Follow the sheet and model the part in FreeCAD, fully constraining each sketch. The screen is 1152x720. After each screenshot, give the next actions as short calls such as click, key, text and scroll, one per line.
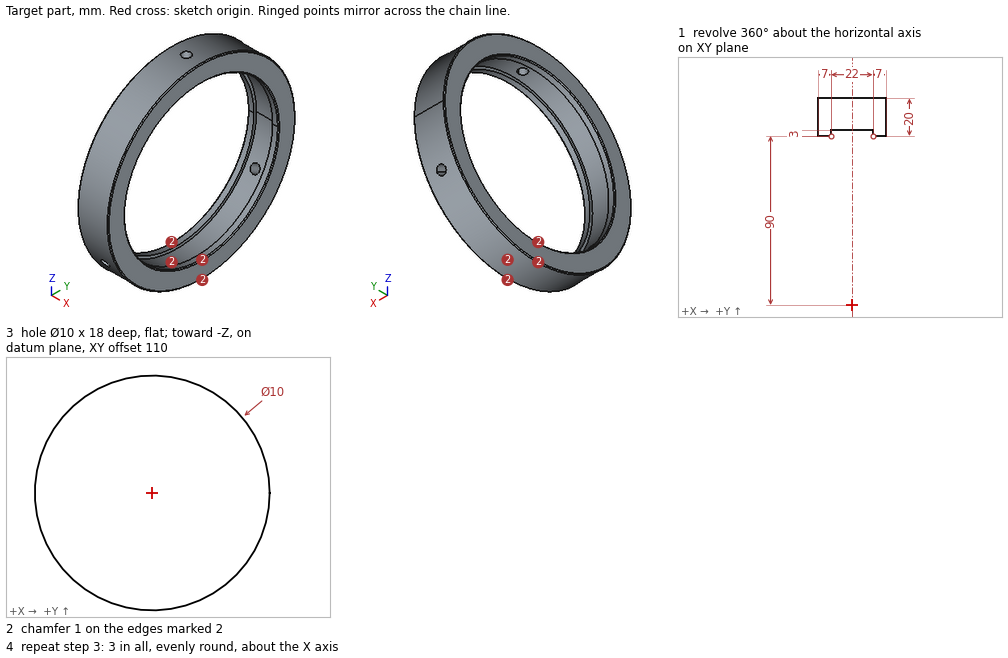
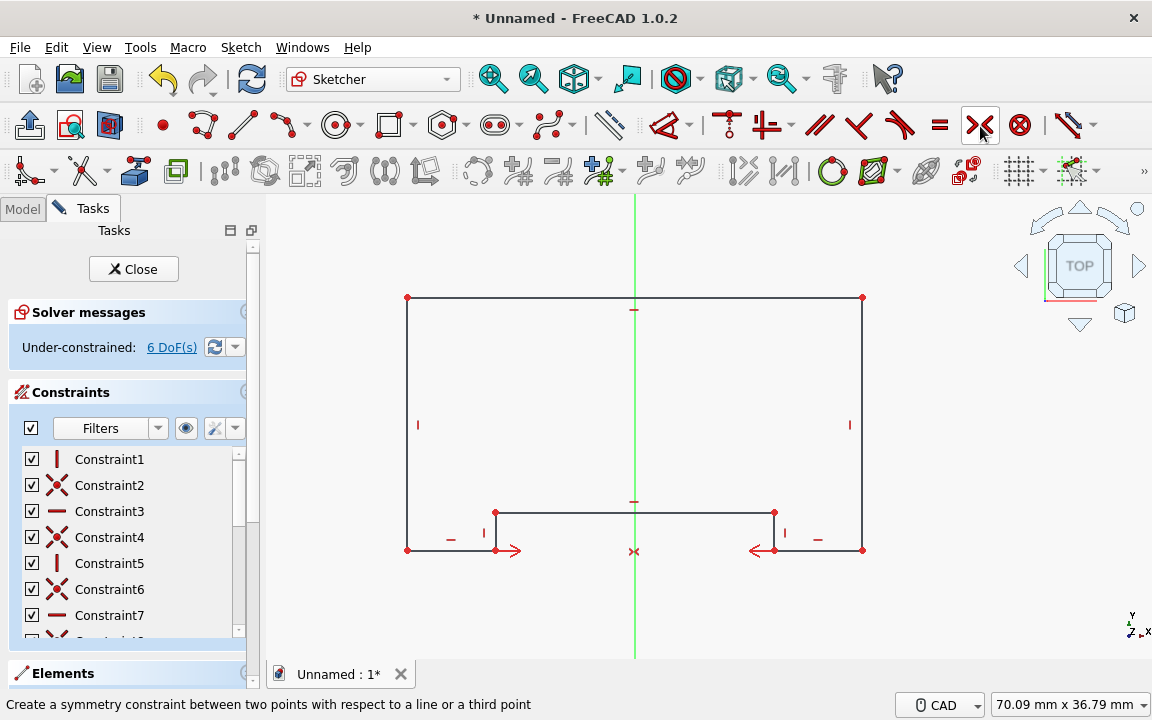
click(496, 540)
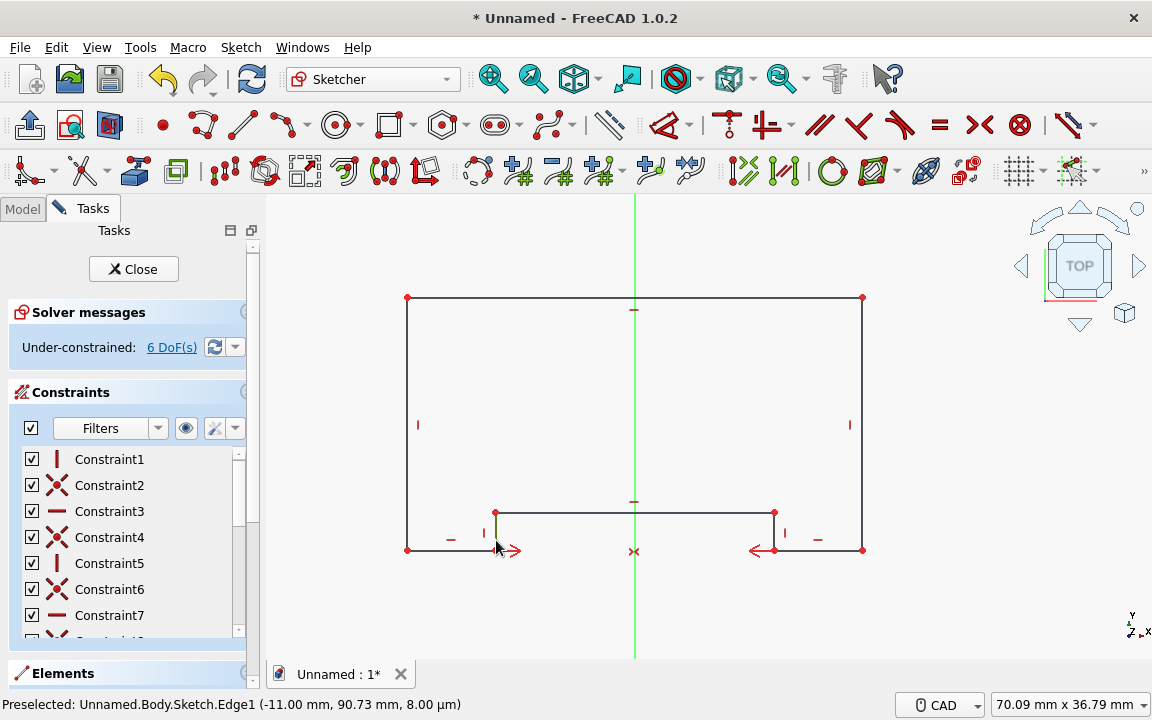
key(i)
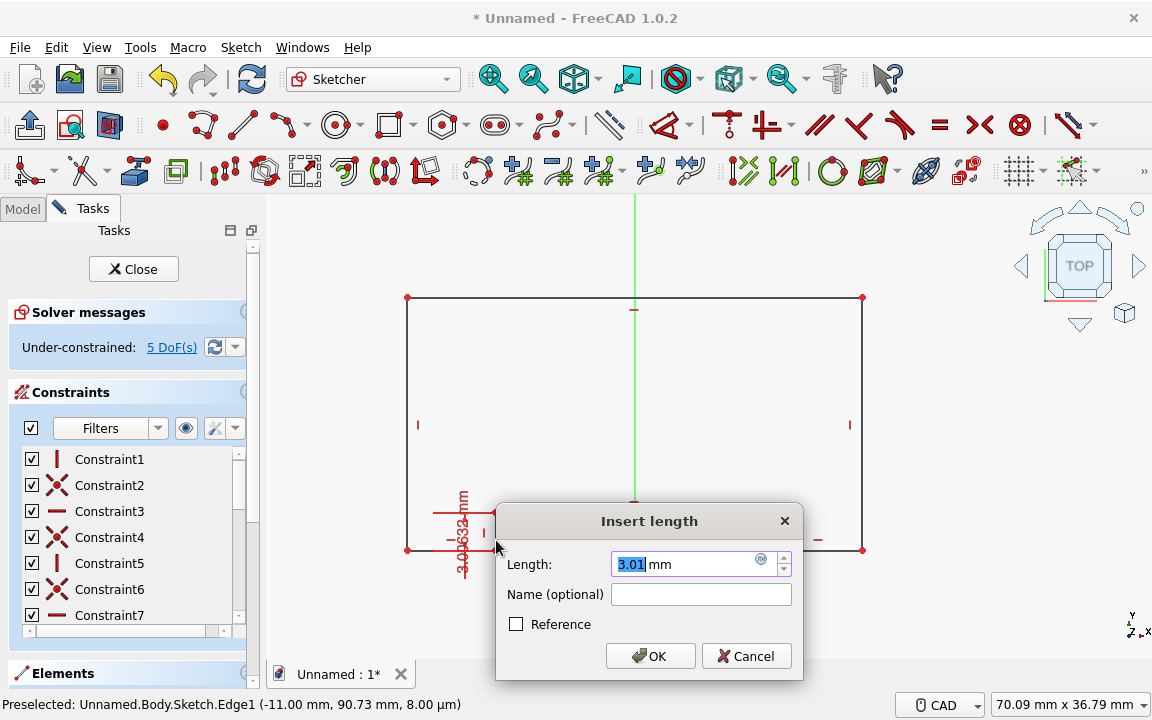
text(3)
key(Return)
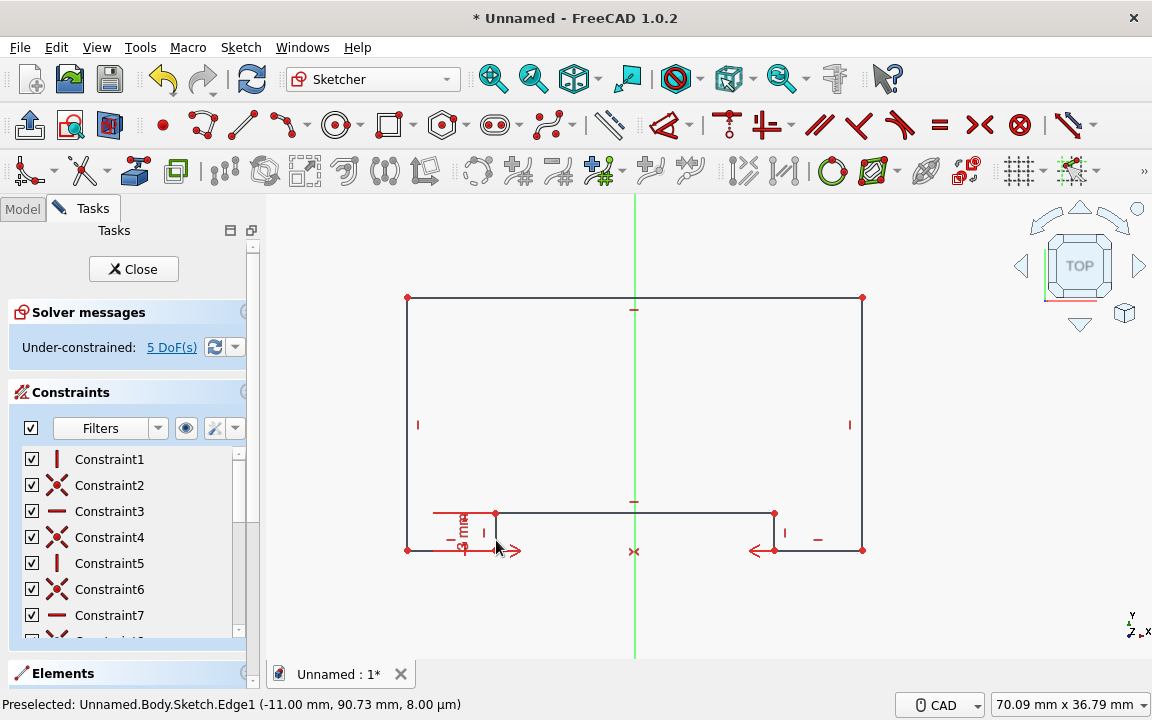
click(800, 551)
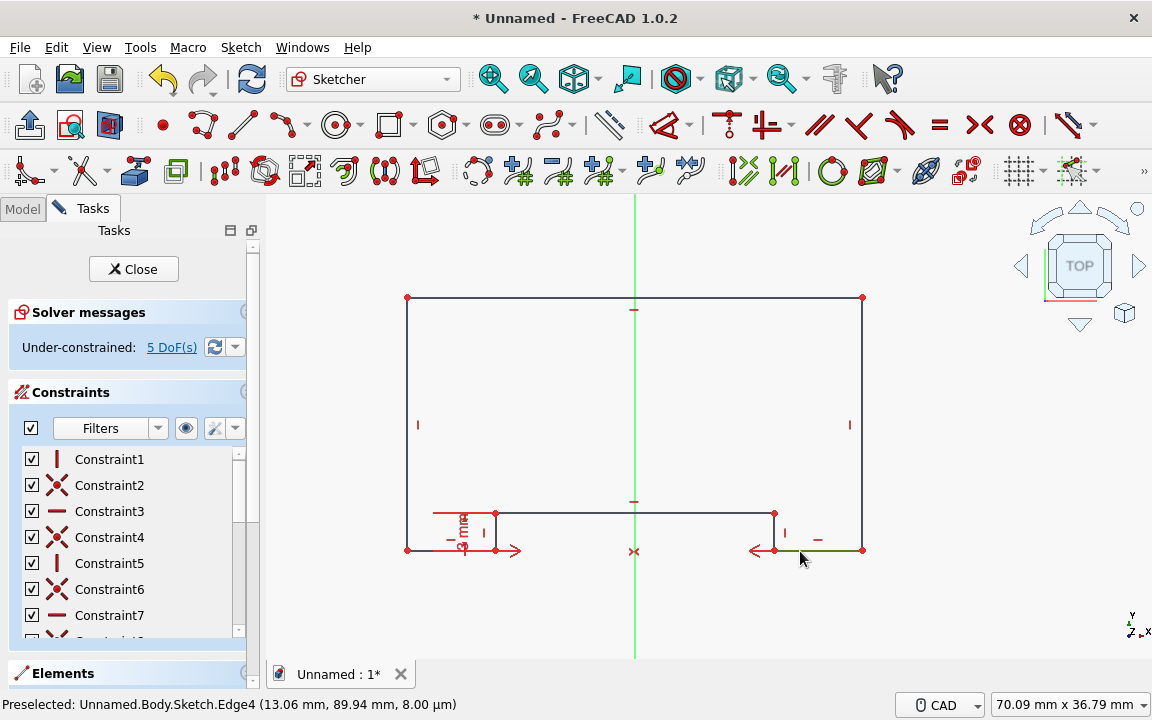
key(l)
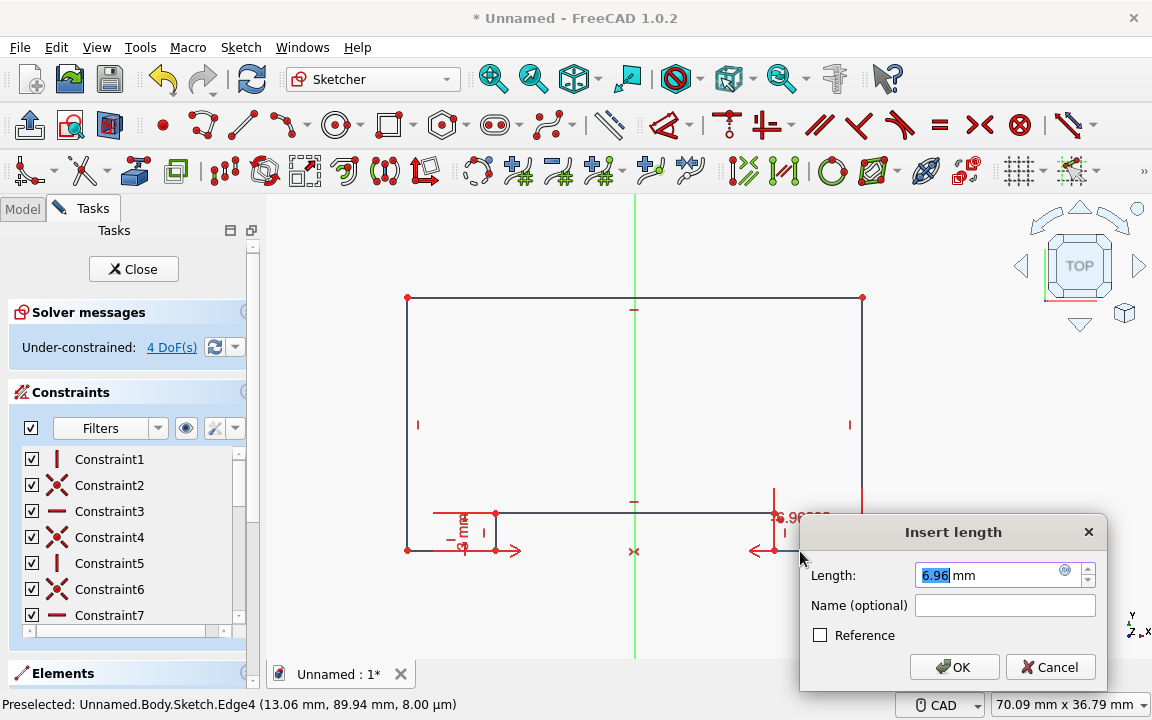
text(7)
key(Return)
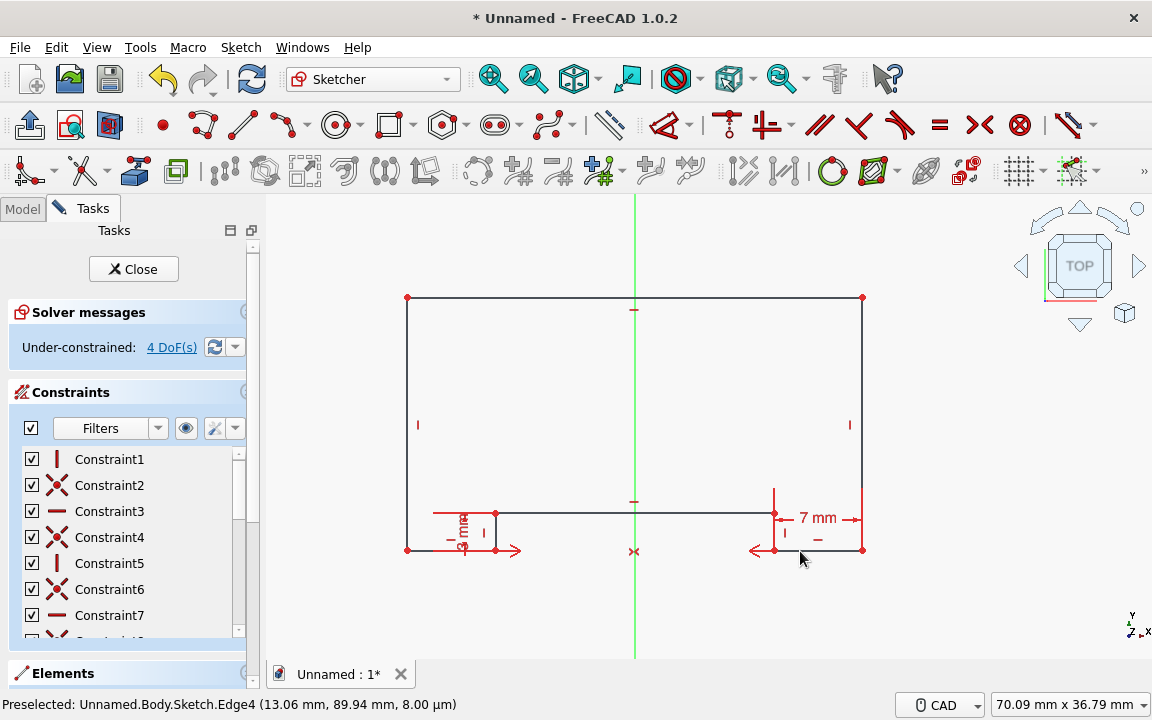
click(434, 551)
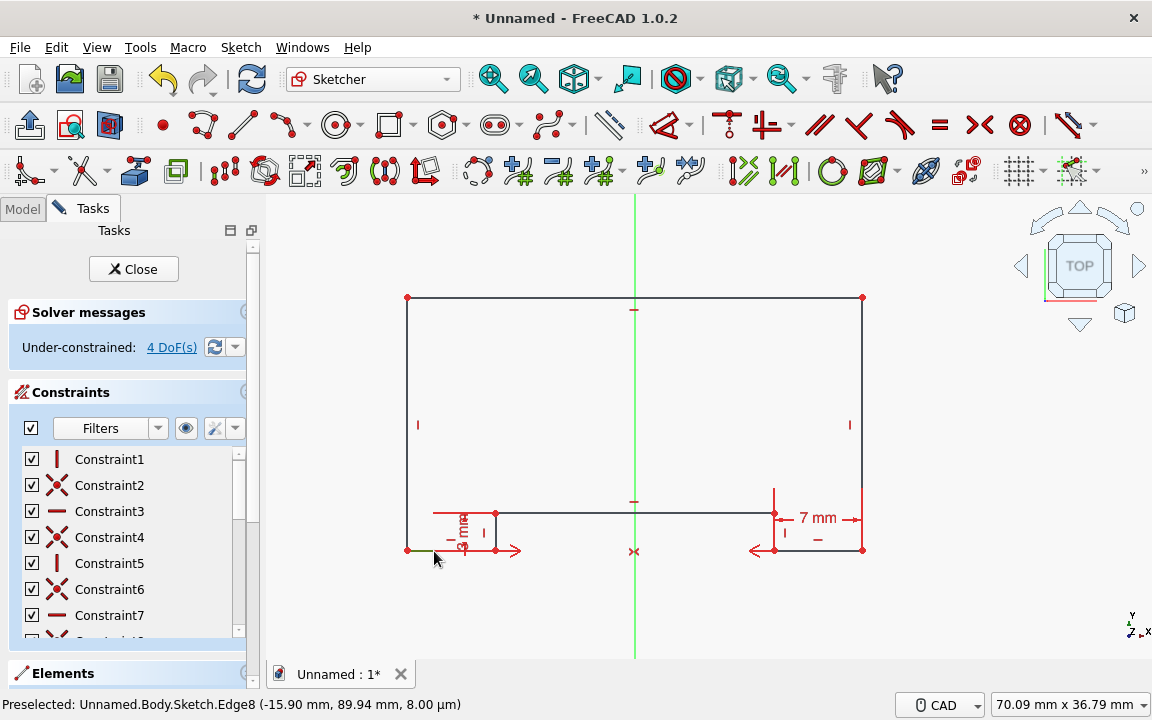
key(l)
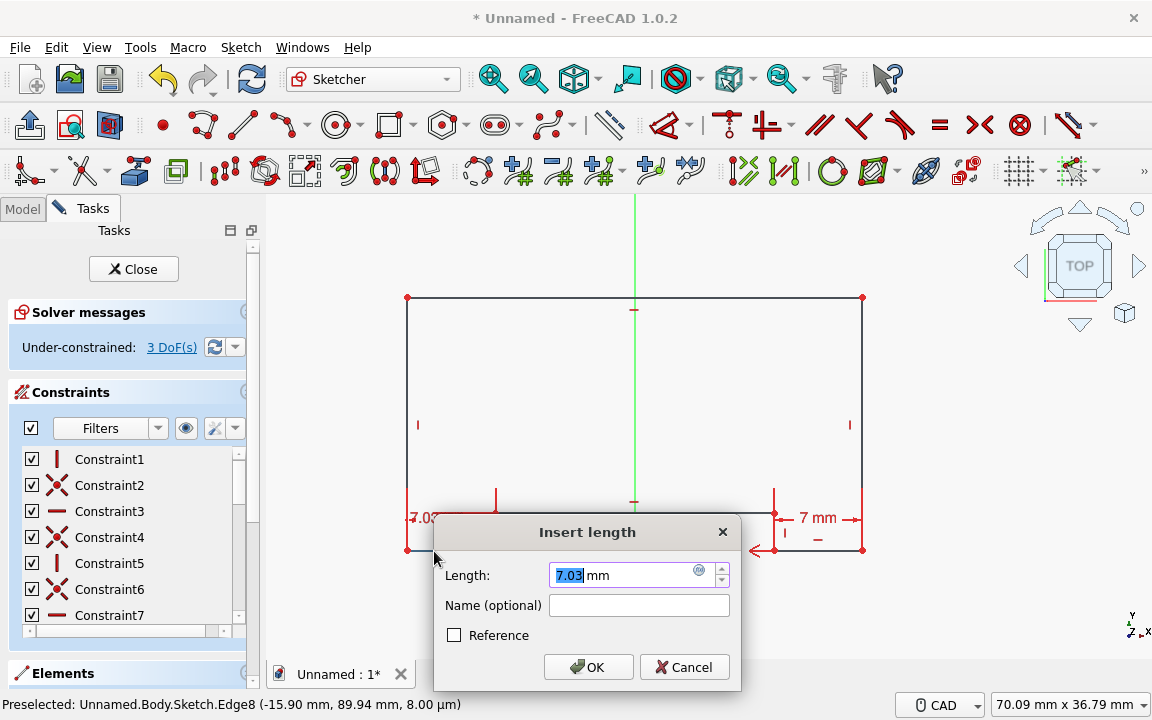
text(7)
key(Return)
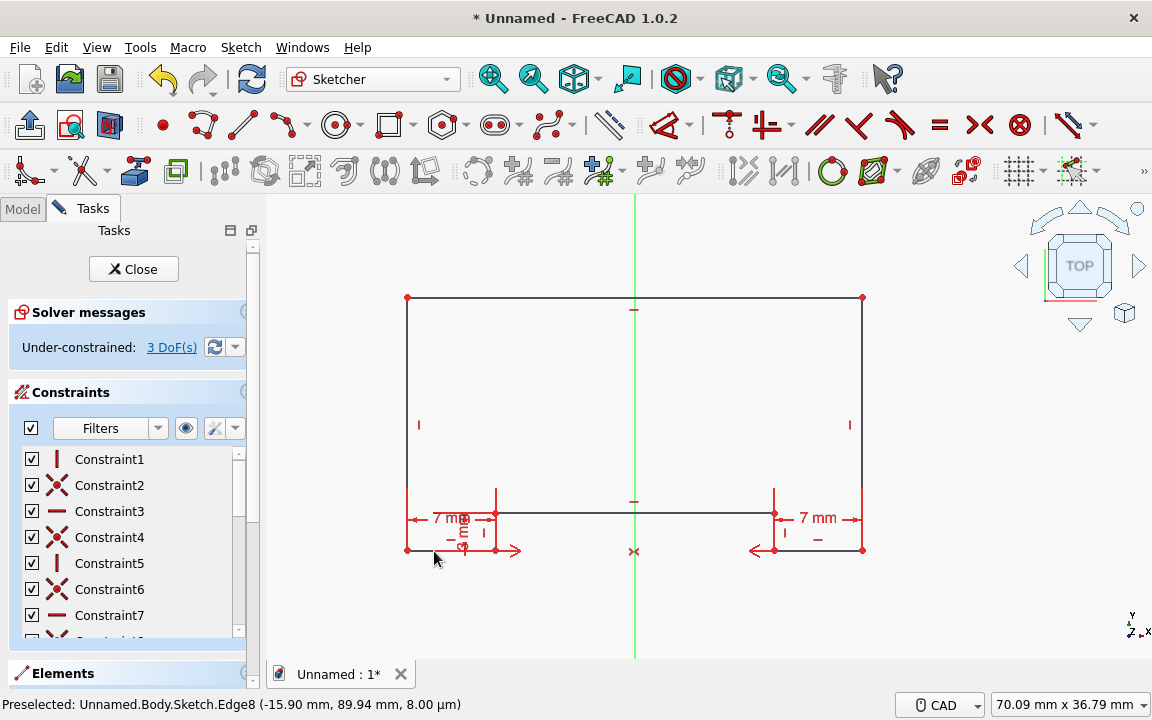
click(579, 513)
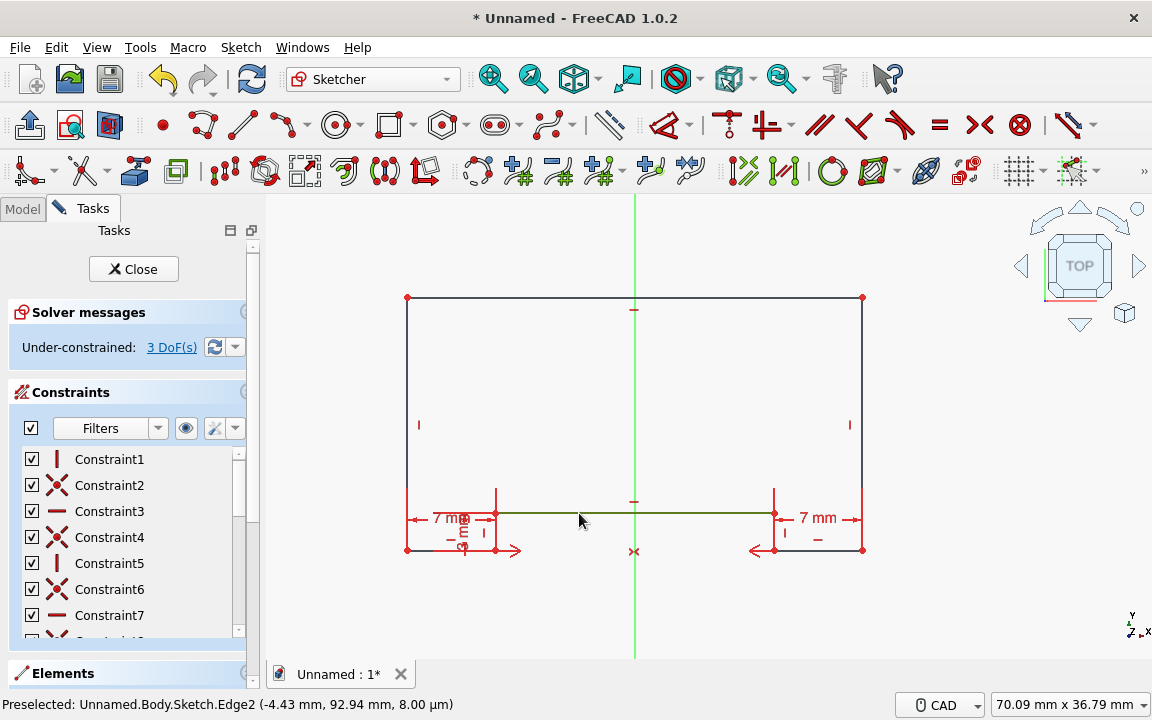
key(l)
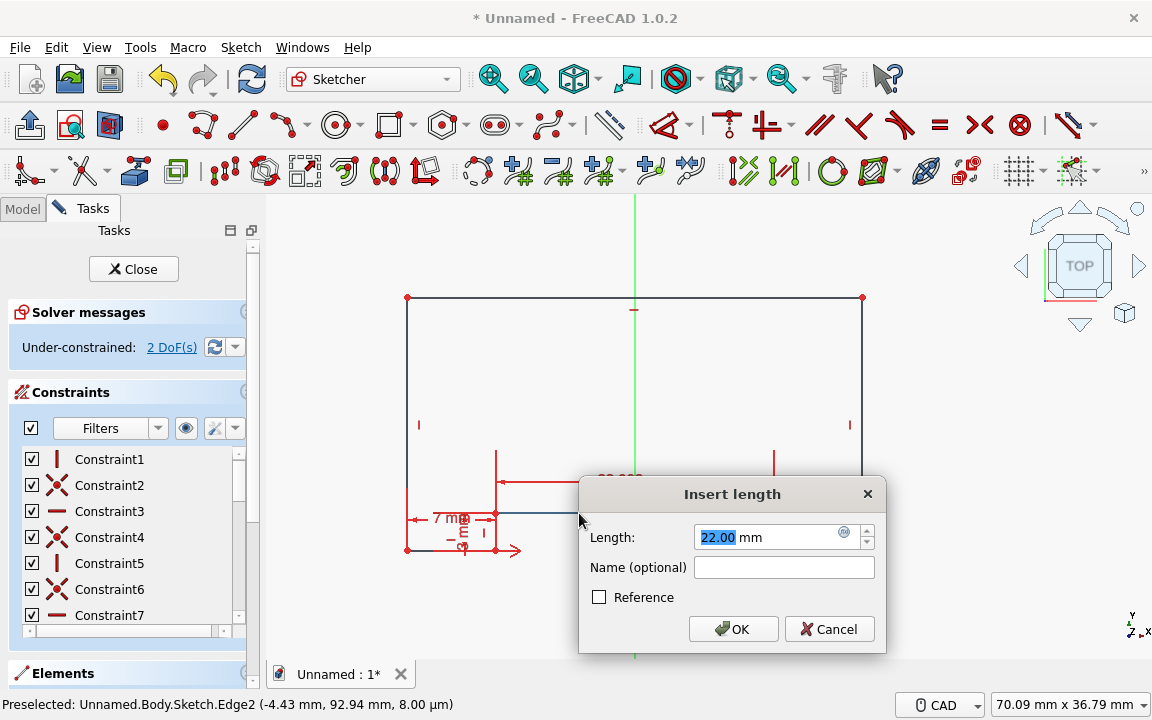
text(22)
key(Return)